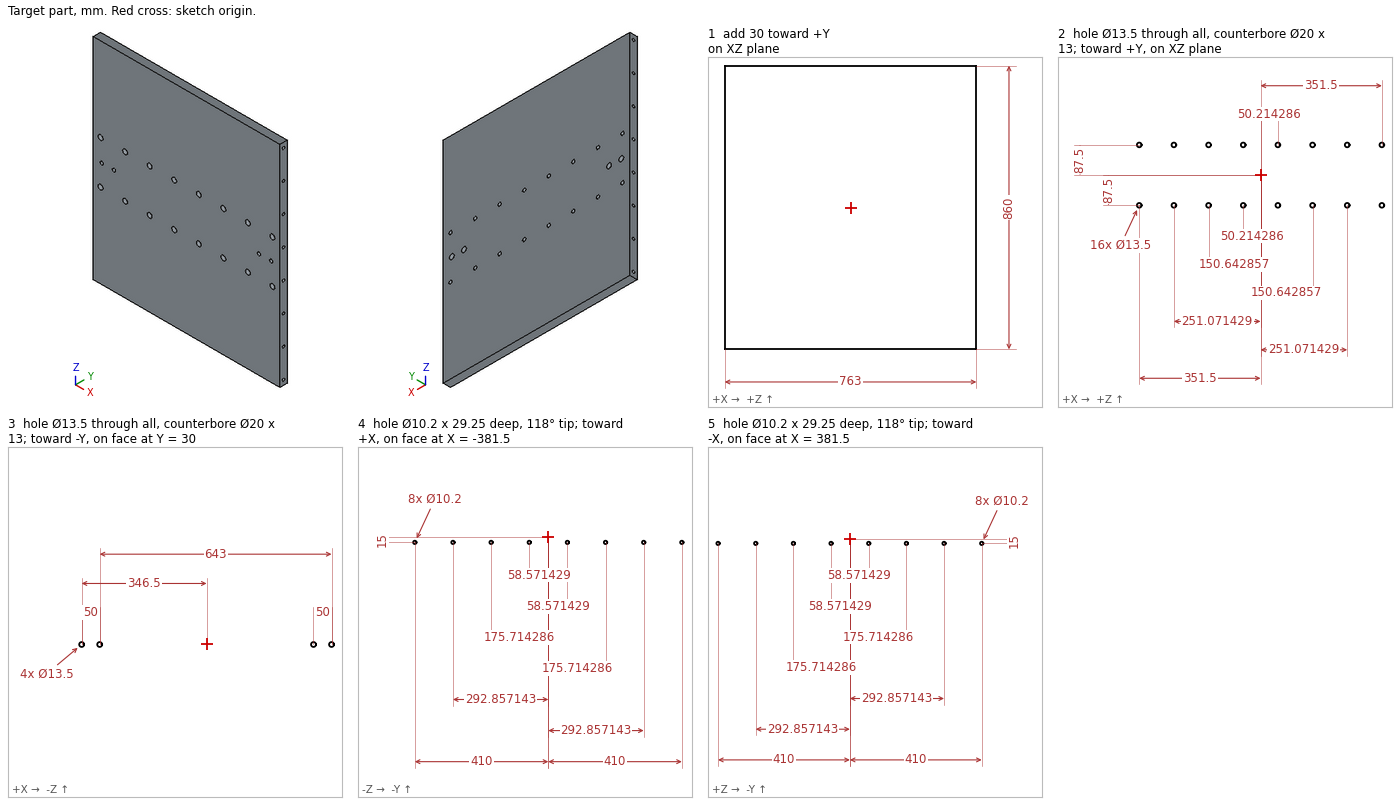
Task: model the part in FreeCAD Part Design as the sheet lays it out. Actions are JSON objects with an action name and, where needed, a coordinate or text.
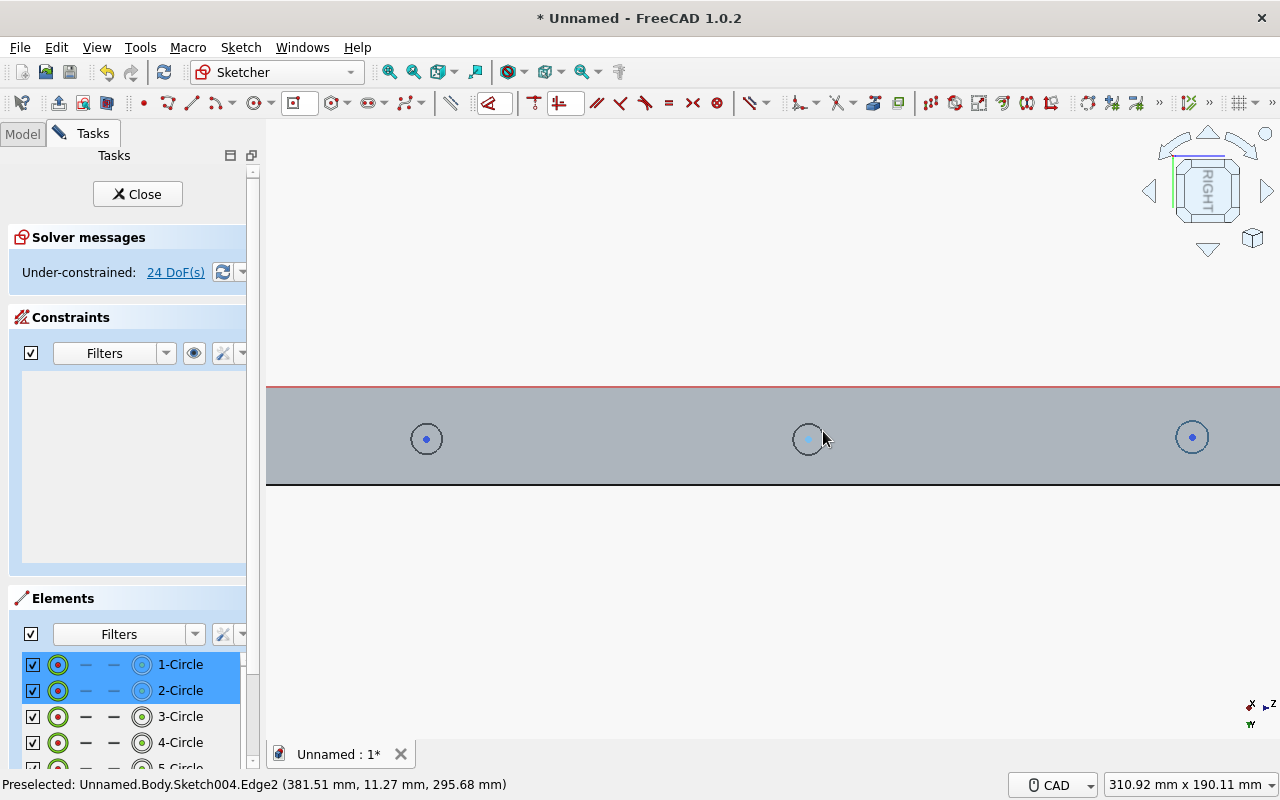
{"action": "left_click", "coordinate": [820, 428]}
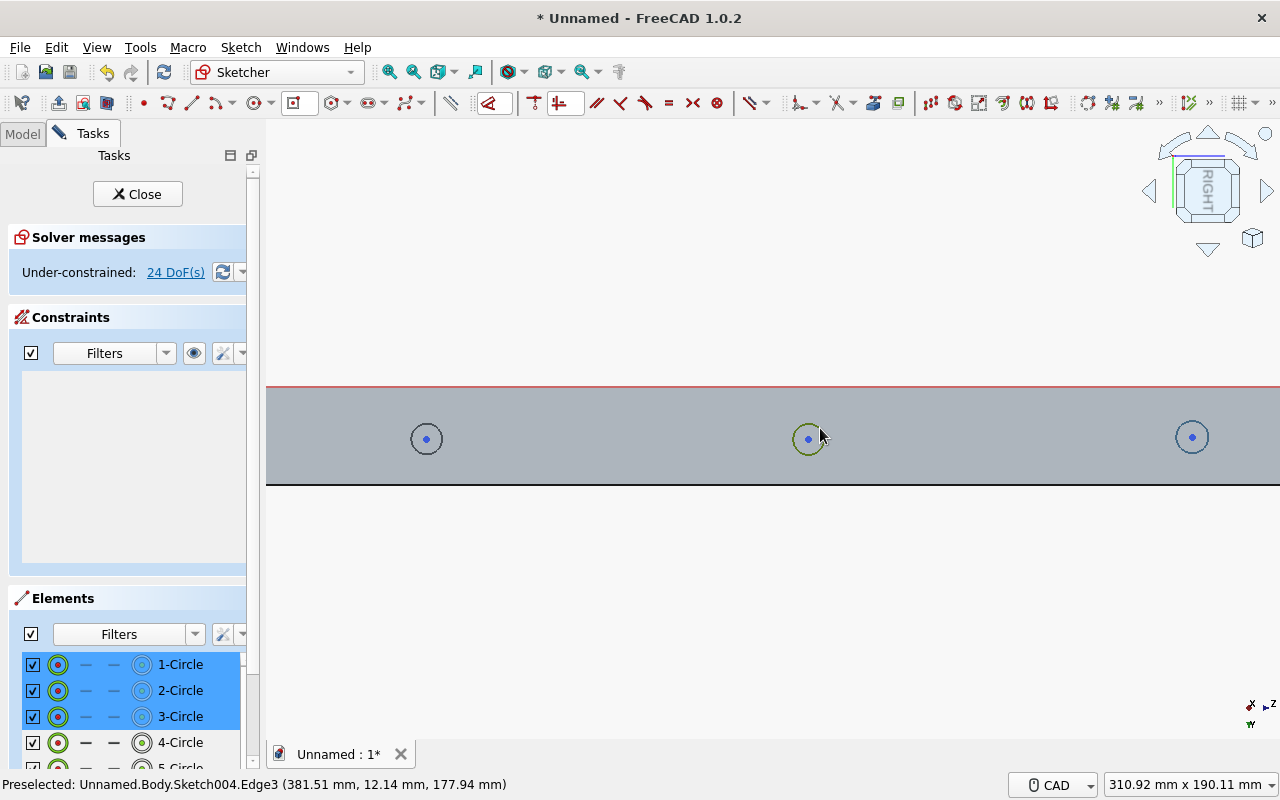
{"action": "left_click", "coordinate": [438, 428]}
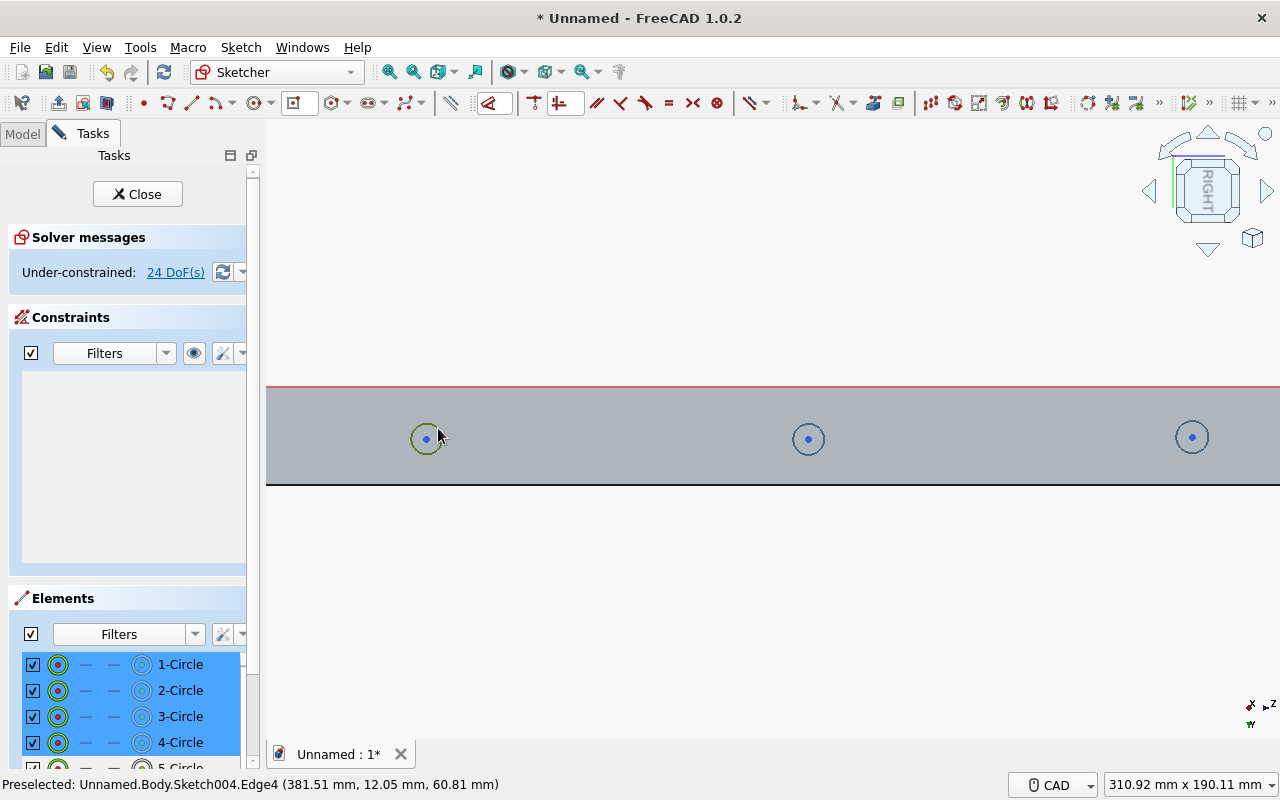
{"action": "scroll", "coordinate": [823, 431], "scroll_direction": "down", "scroll_amount": 8}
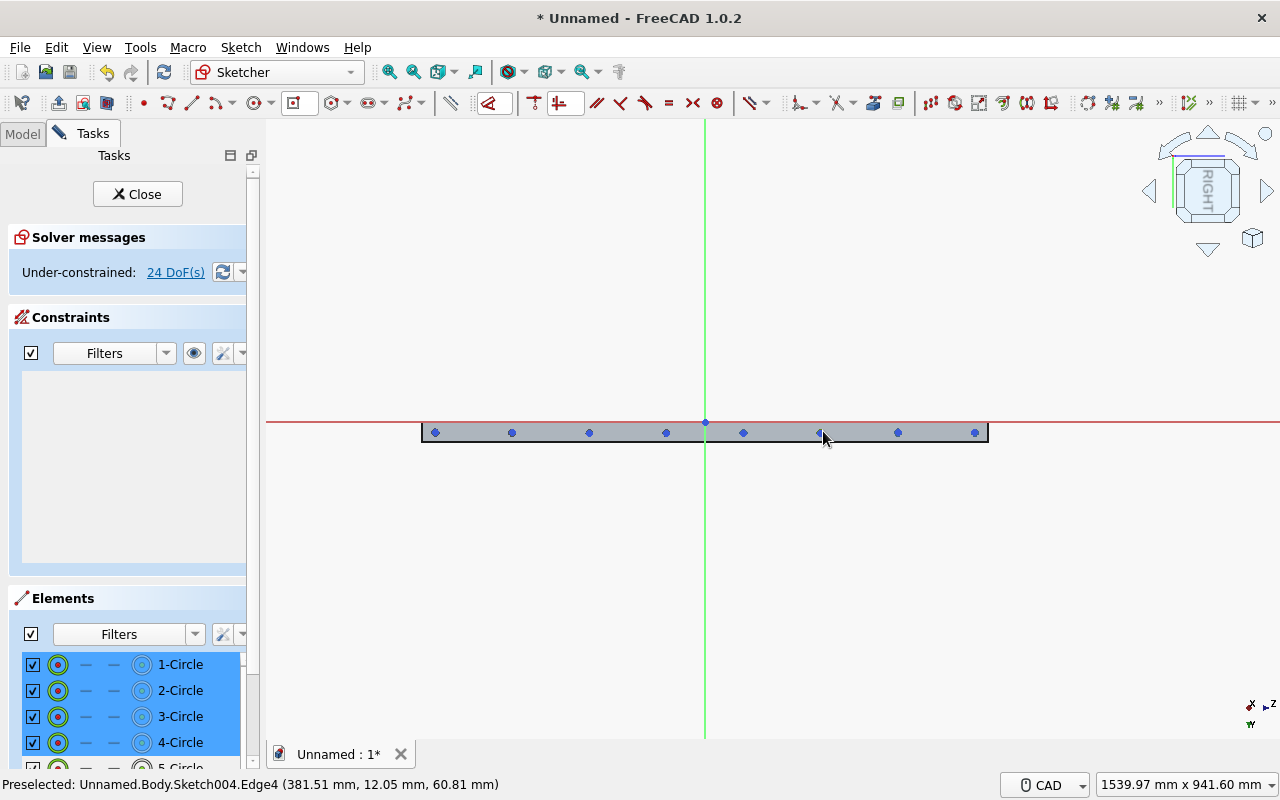
{"action": "scroll", "coordinate": [668, 431], "scroll_direction": "up", "scroll_amount": 8}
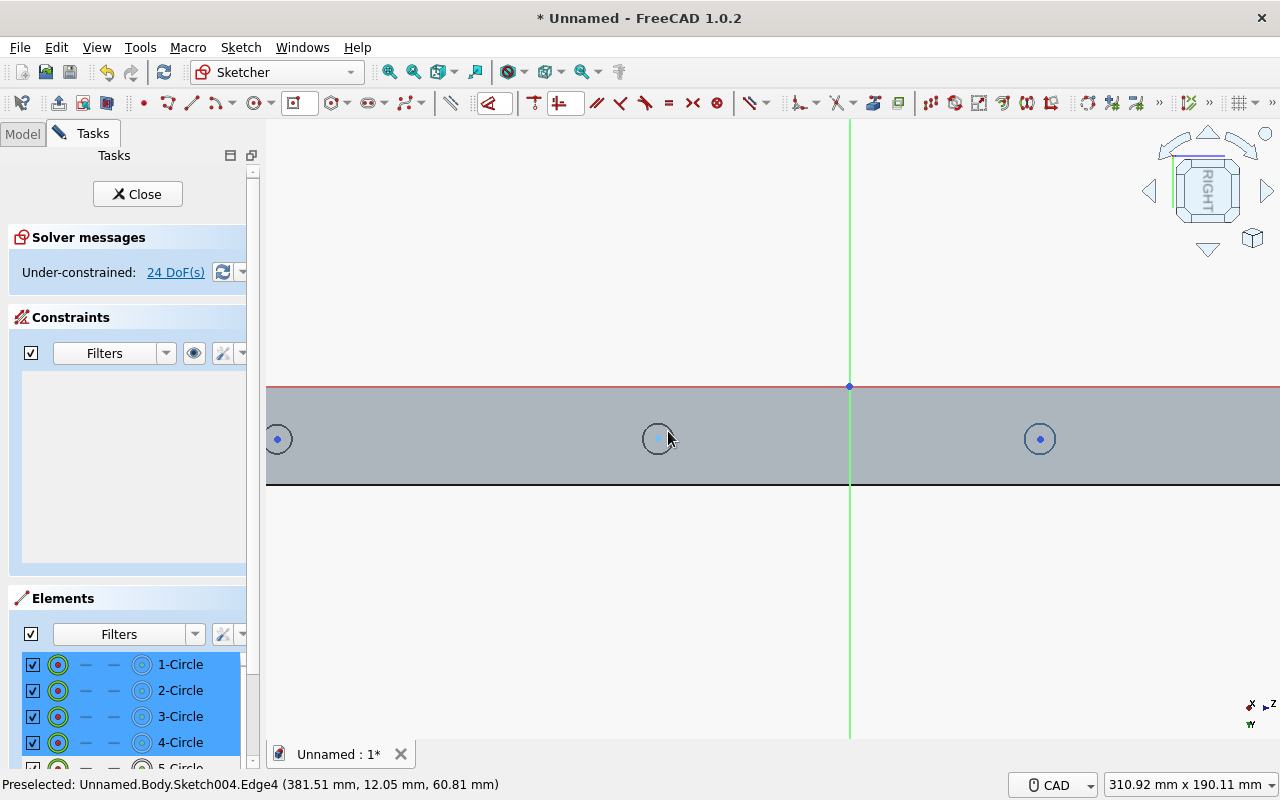
{"action": "left_click", "coordinate": [669, 428]}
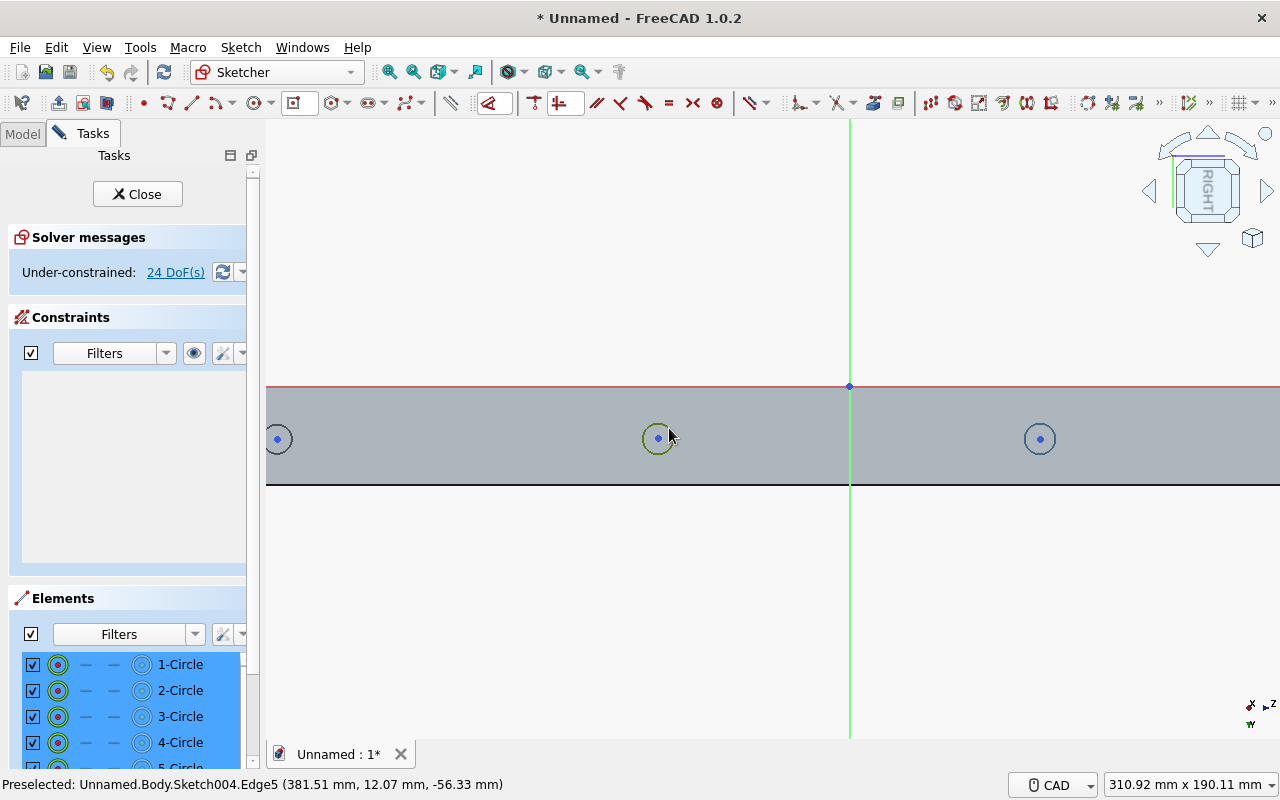
{"action": "scroll", "coordinate": [668, 431], "scroll_direction": "down", "scroll_amount": 8}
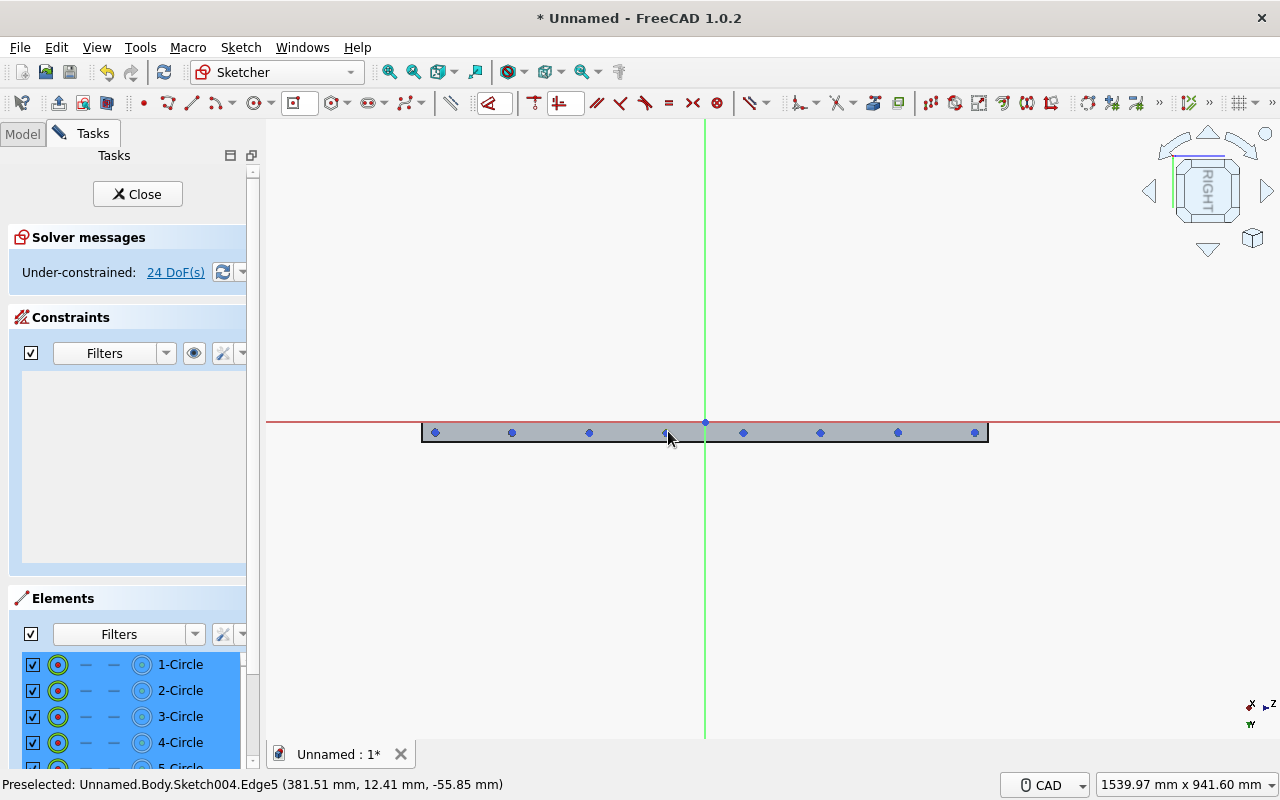
{"action": "scroll", "coordinate": [591, 431], "scroll_direction": "up", "scroll_amount": 8}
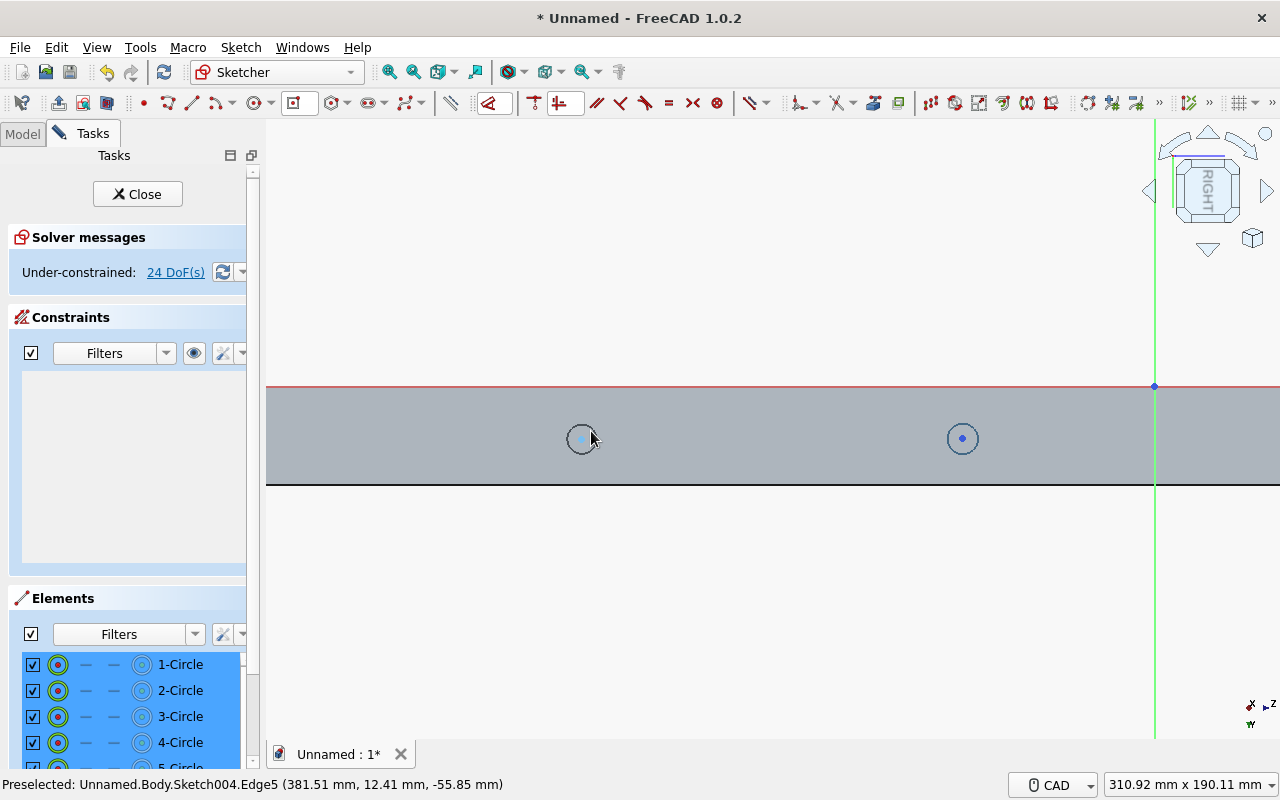
{"action": "left_click", "coordinate": [592, 429]}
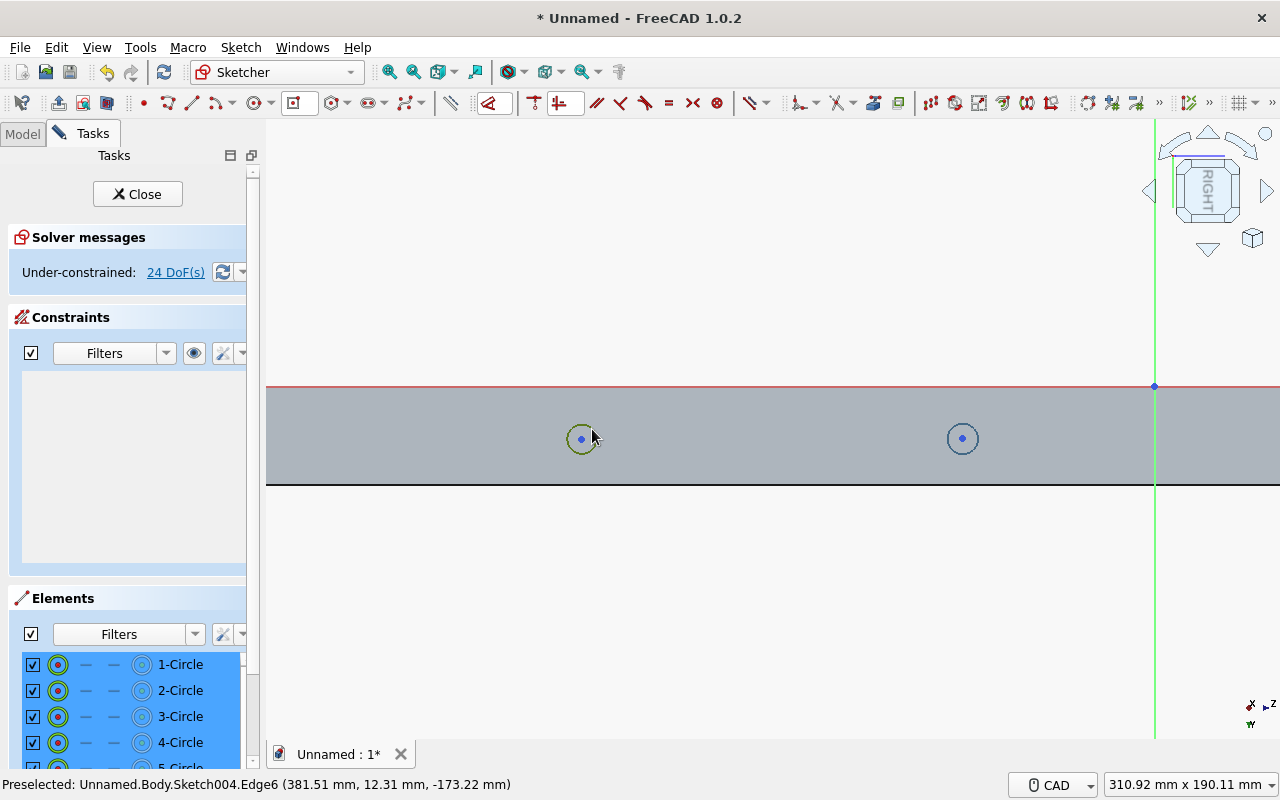
{"action": "scroll", "coordinate": [591, 431], "scroll_direction": "down", "scroll_amount": 8}